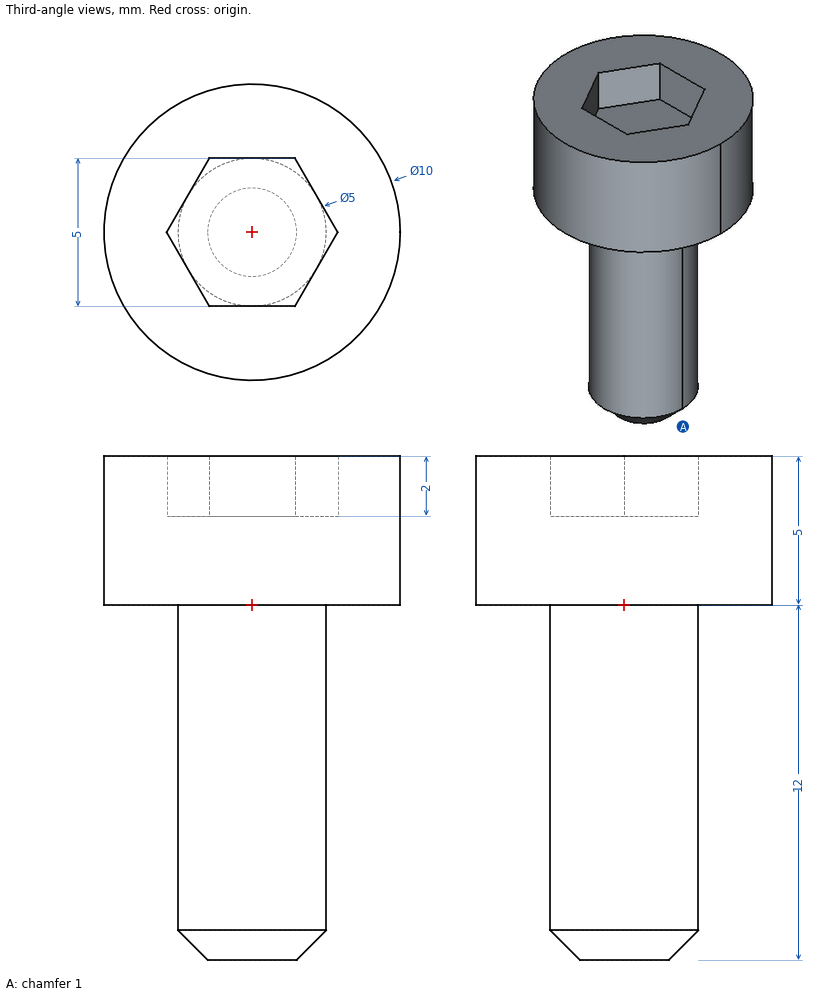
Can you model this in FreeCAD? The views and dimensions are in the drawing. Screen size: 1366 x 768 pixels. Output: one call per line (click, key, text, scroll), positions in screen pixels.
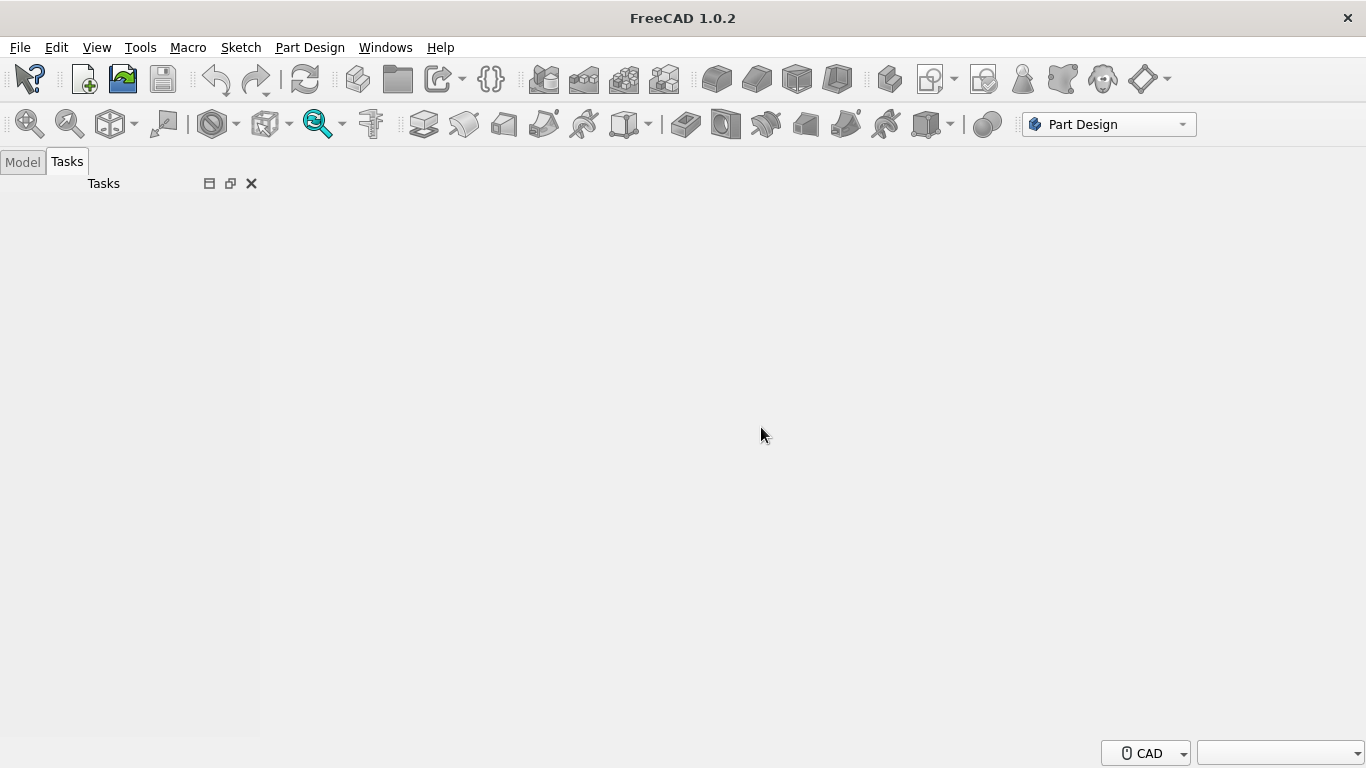
click(84, 80)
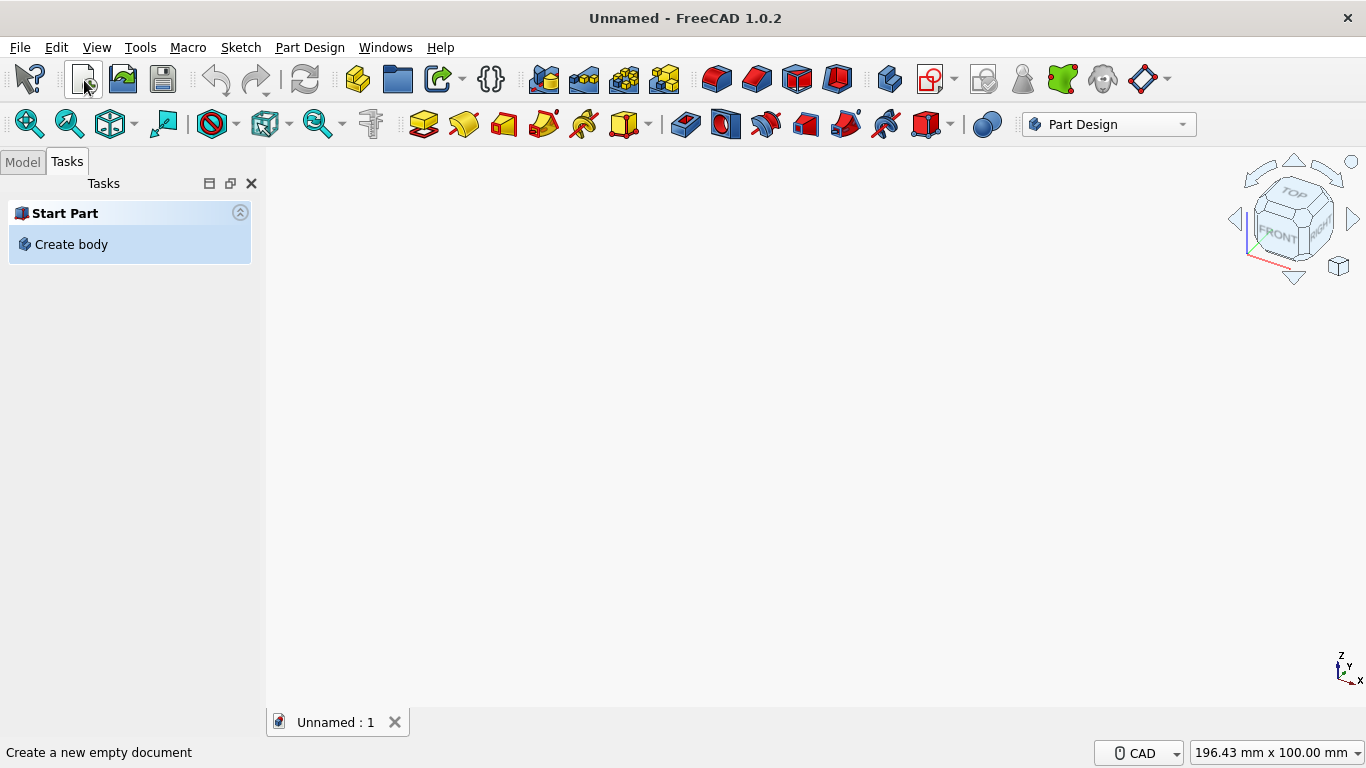
click(930, 80)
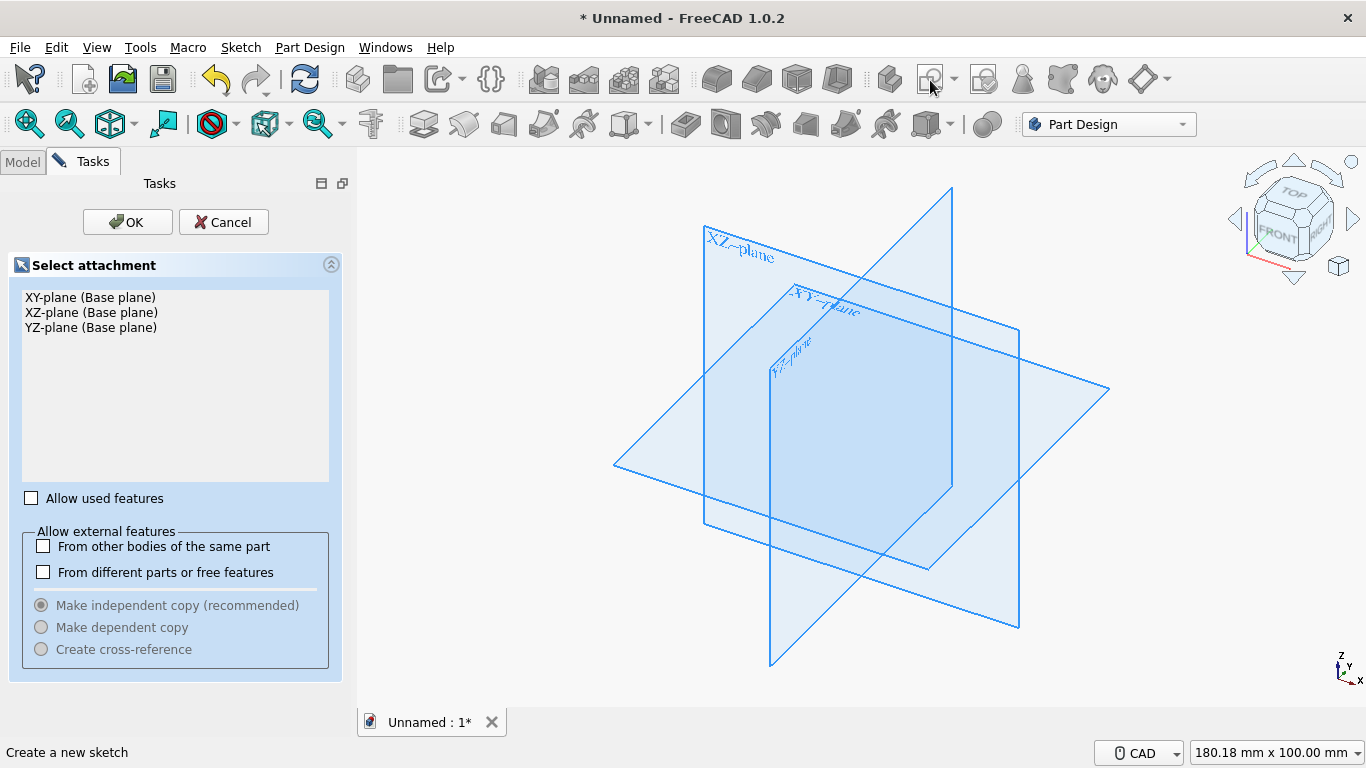
click(82, 298)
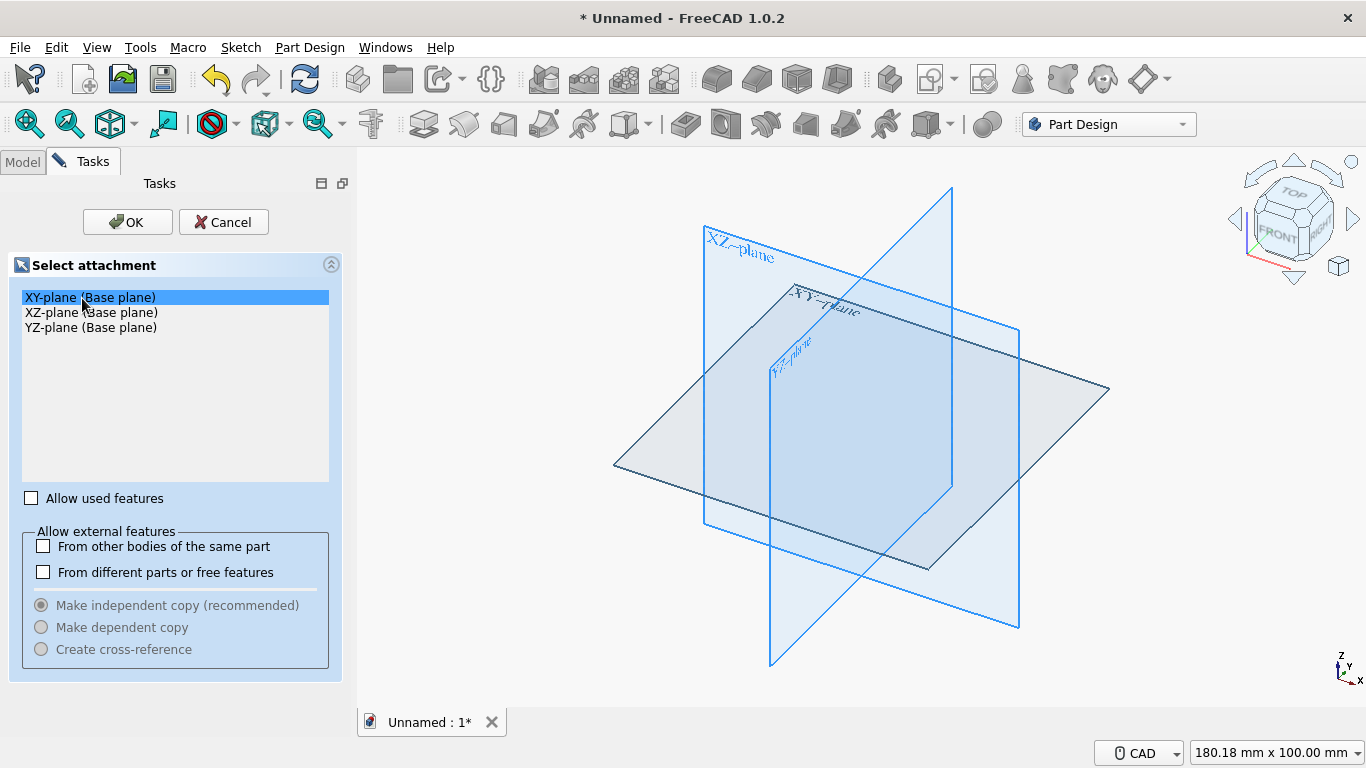
click(128, 222)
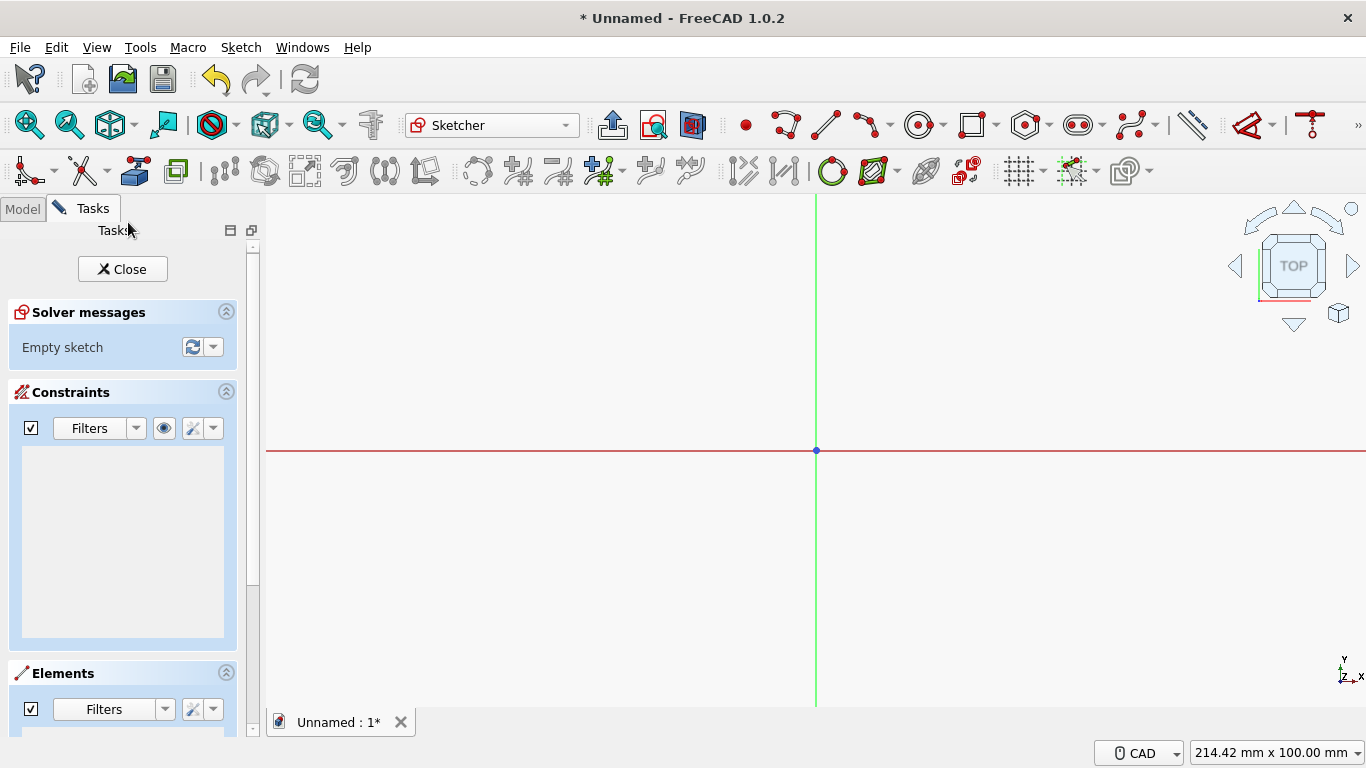
scroll(830, 451, up, 9)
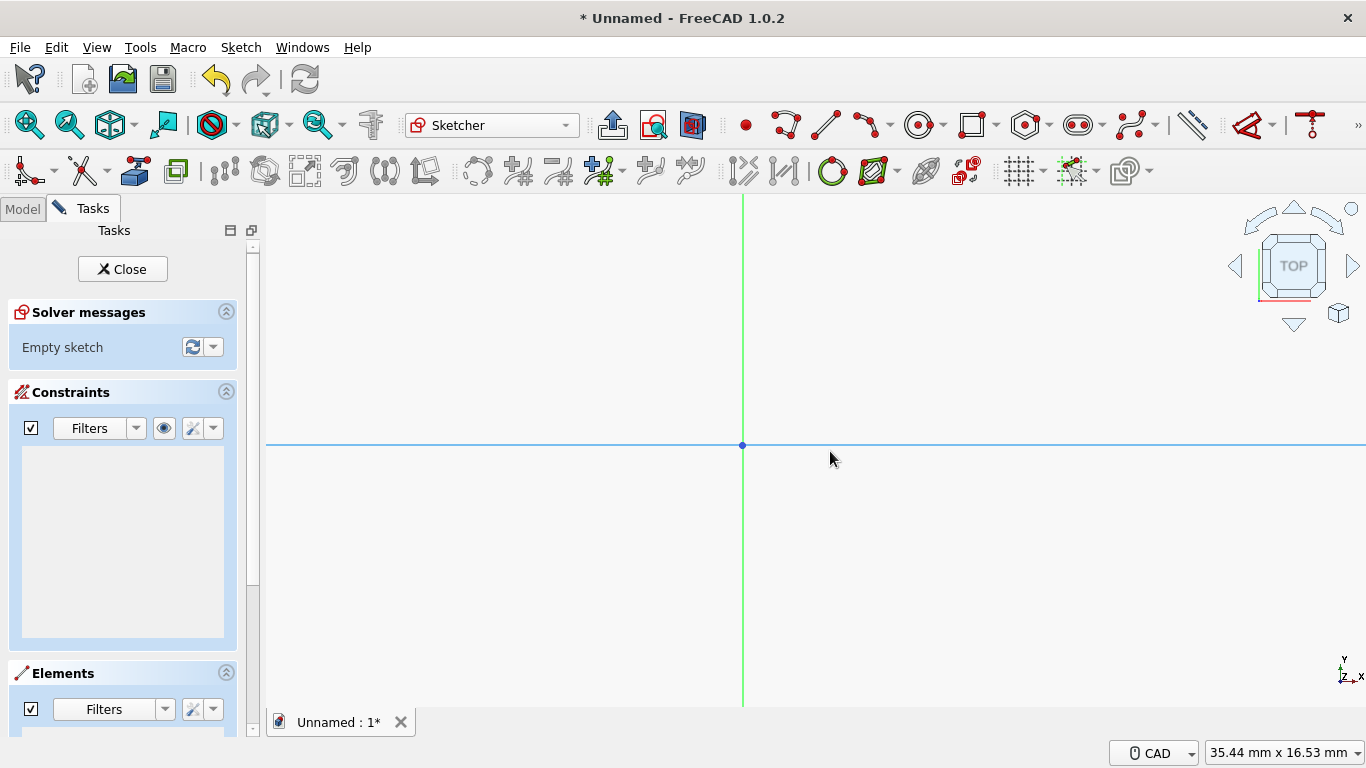
key(g)
key(c)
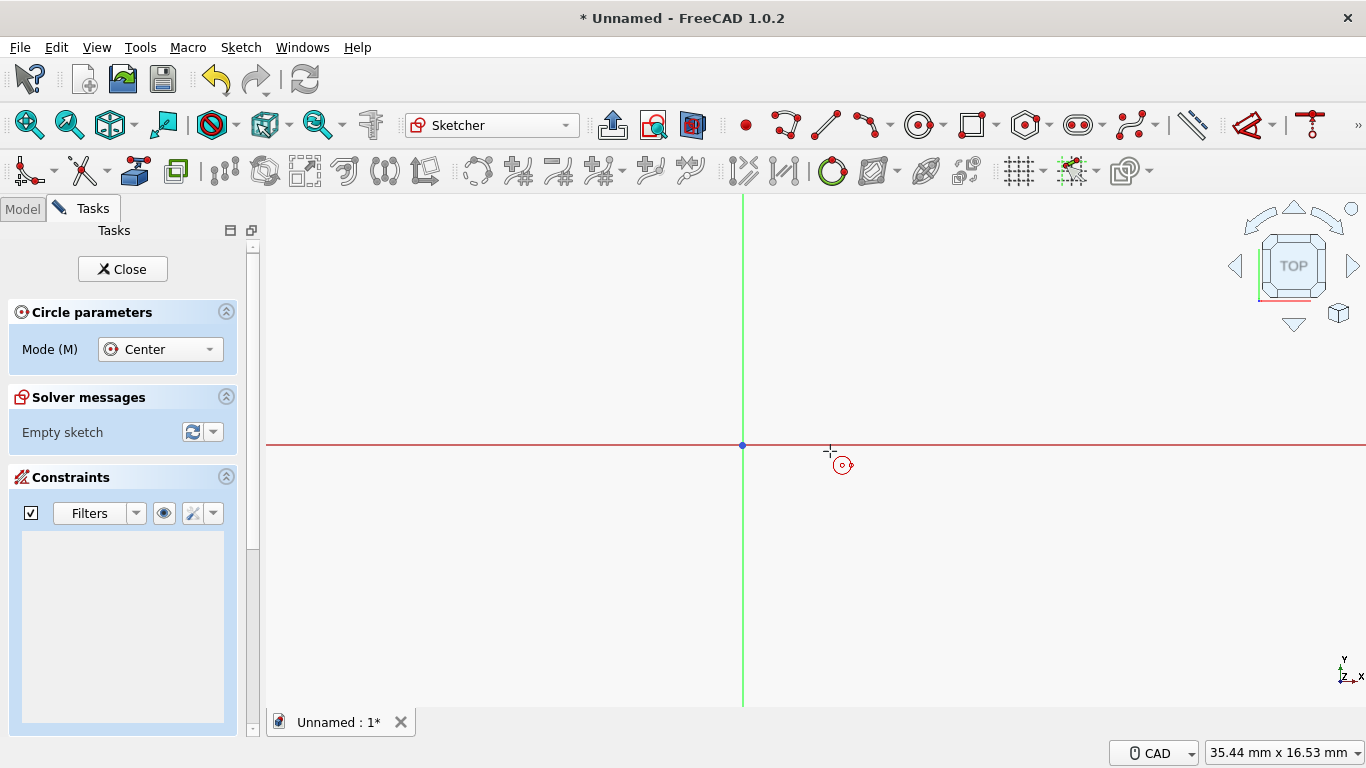
click(743, 445)
click(852, 336)
key(Escape)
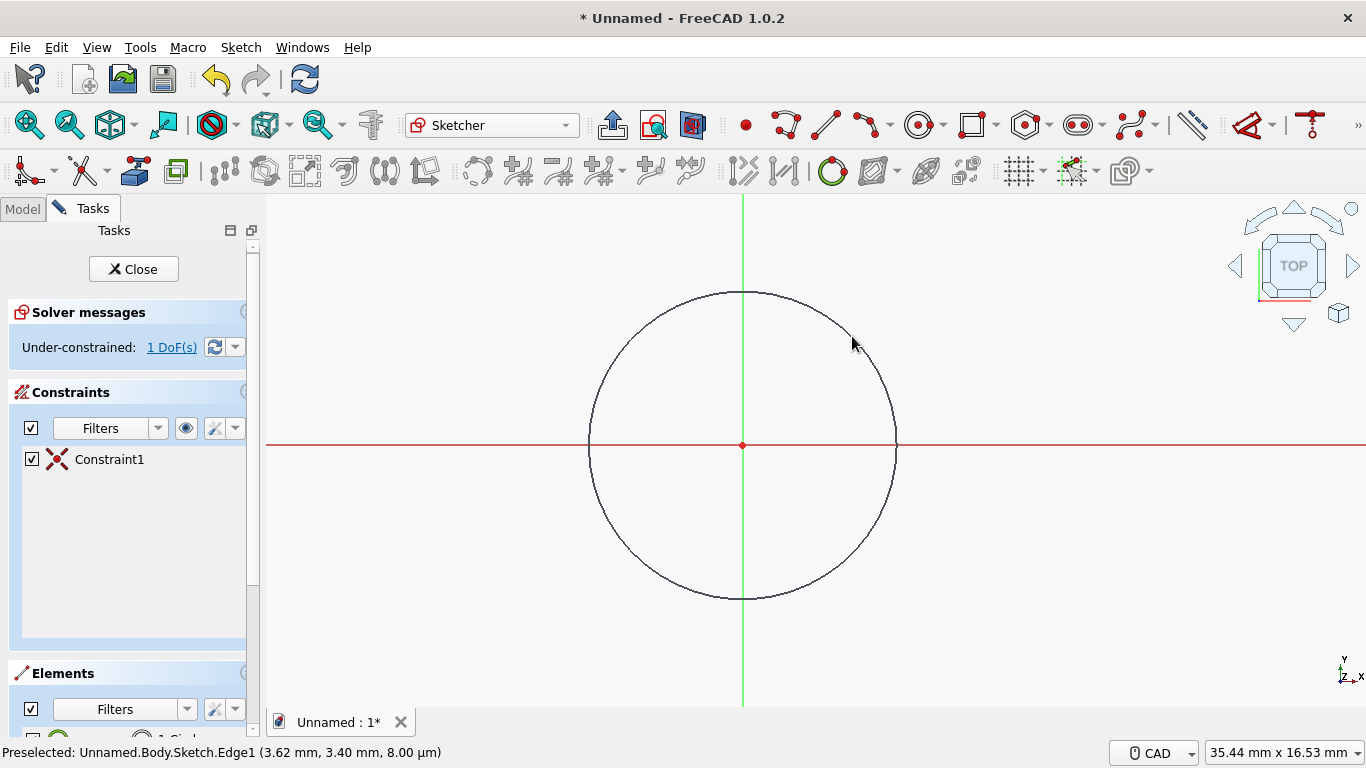
click(1248, 126)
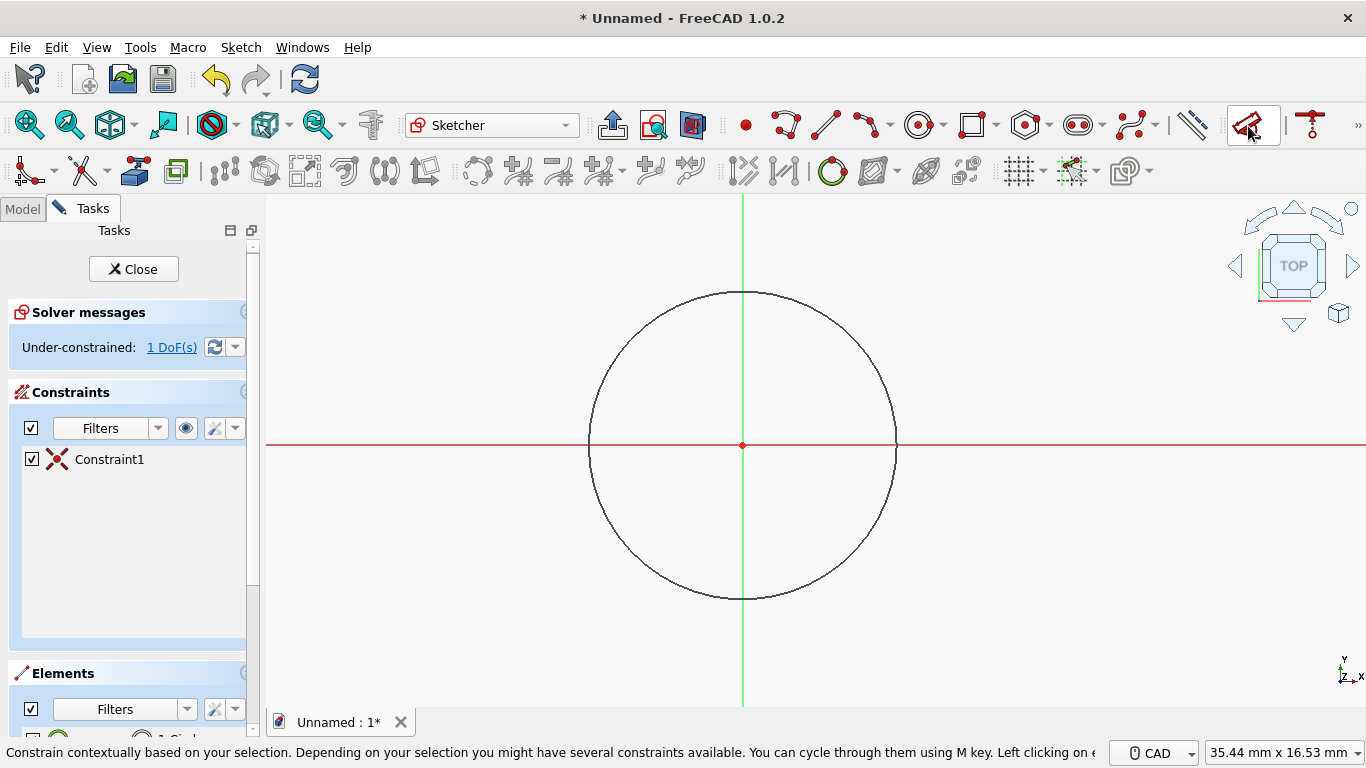
click(851, 336)
click(874, 313)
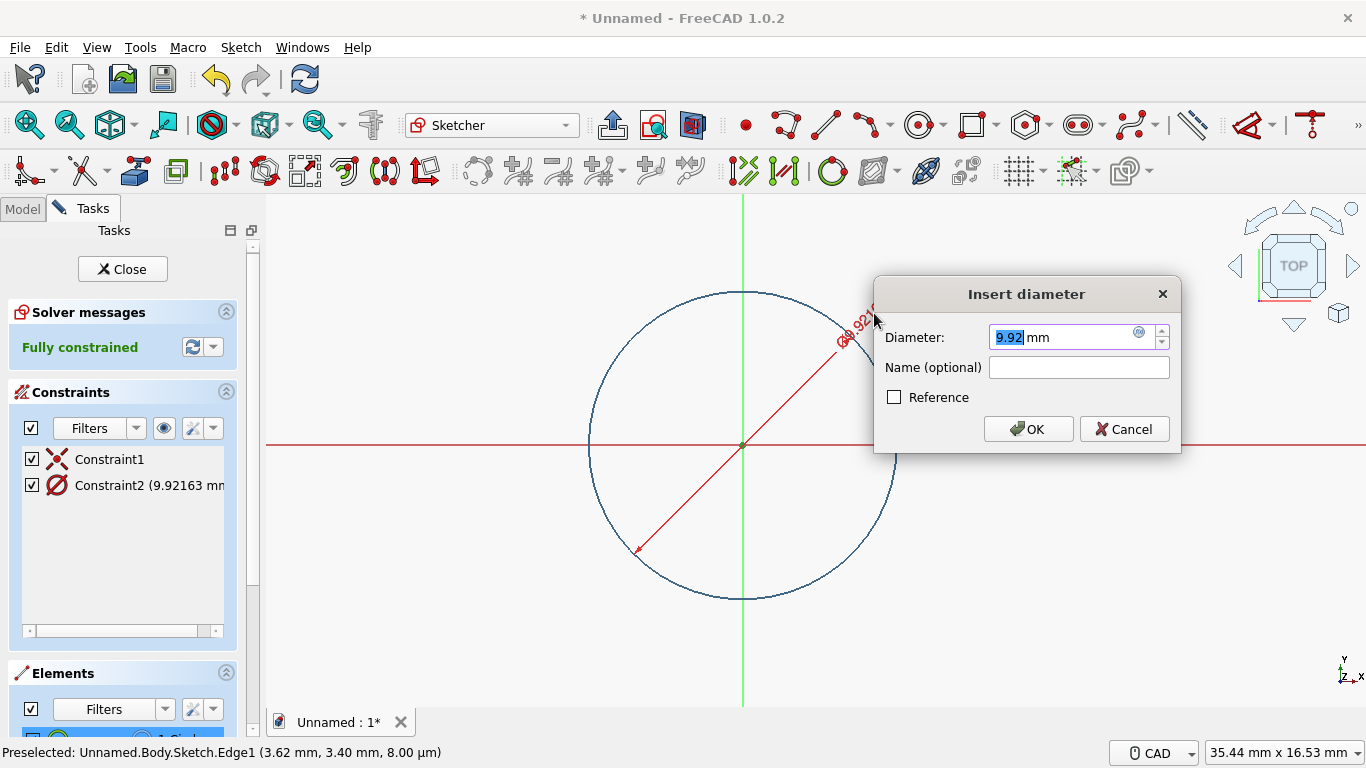
text(10)
key(Return)
key(Escape)